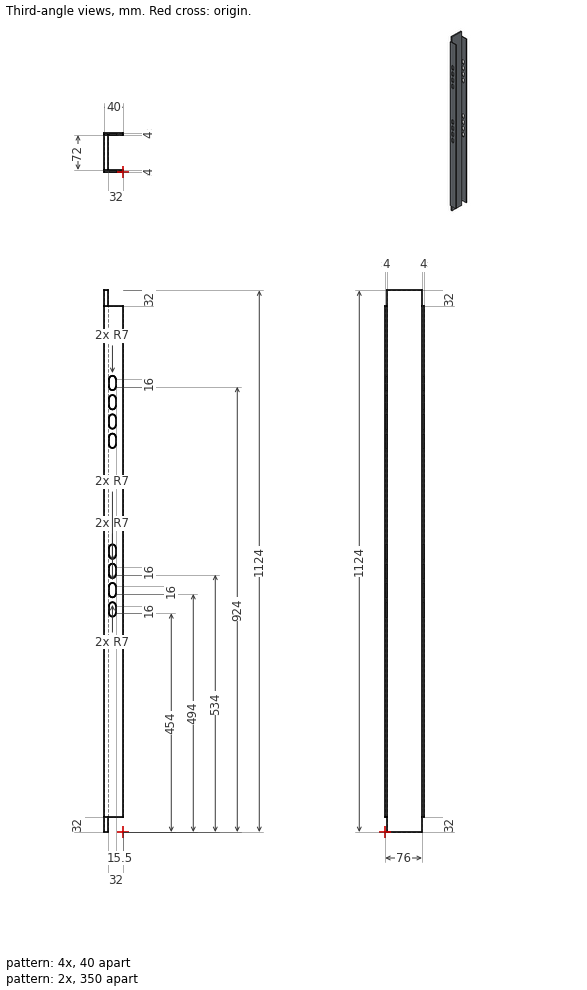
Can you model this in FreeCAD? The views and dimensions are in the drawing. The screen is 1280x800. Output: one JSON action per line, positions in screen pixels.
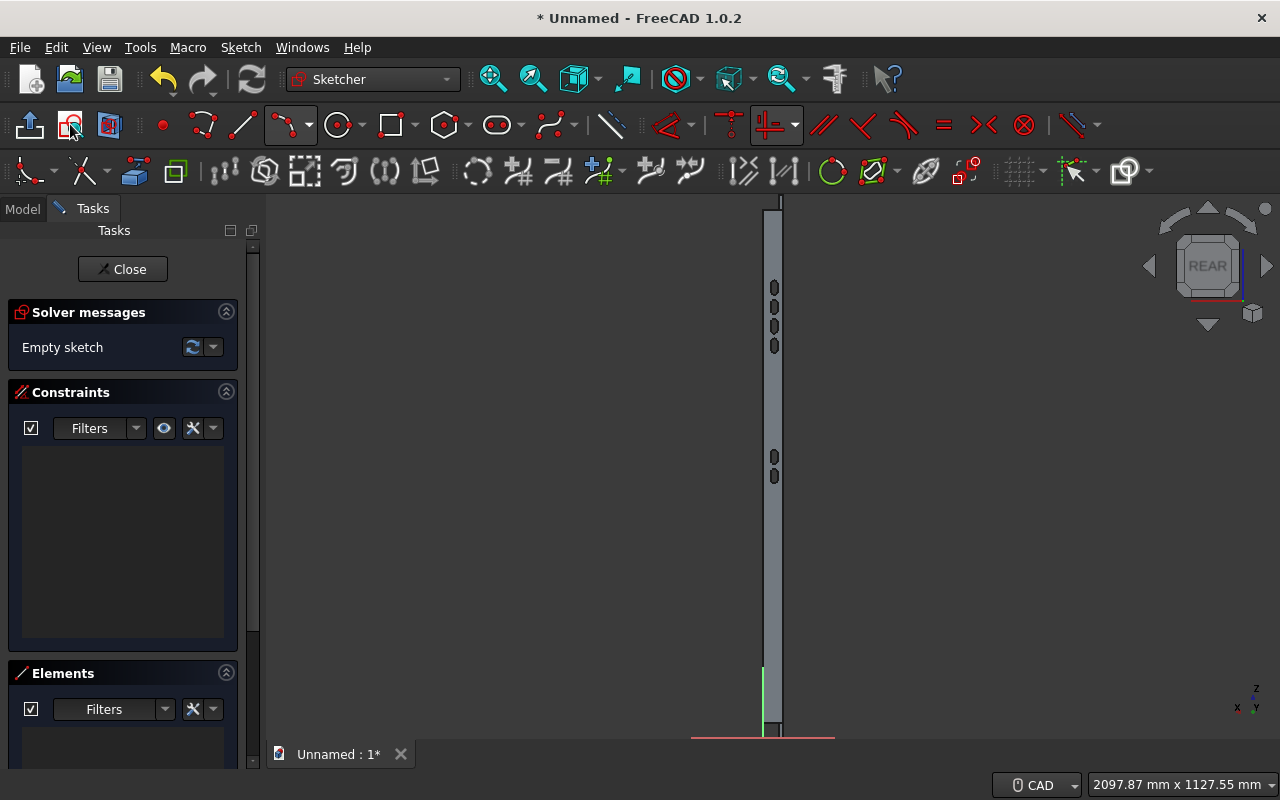
{"action": "scroll", "coordinate": [778, 497], "scroll_direction": "up", "scroll_amount": 15}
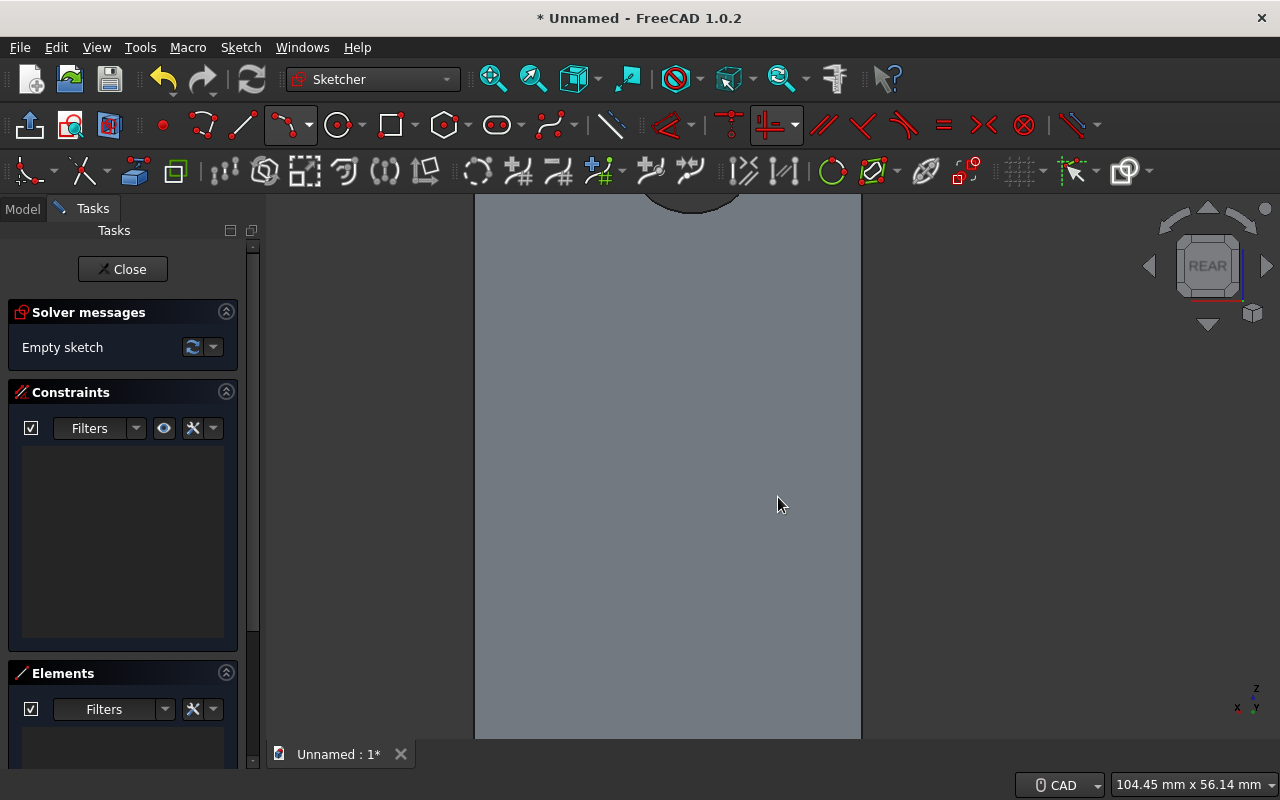
{"action": "left_click", "coordinate": [498, 126]}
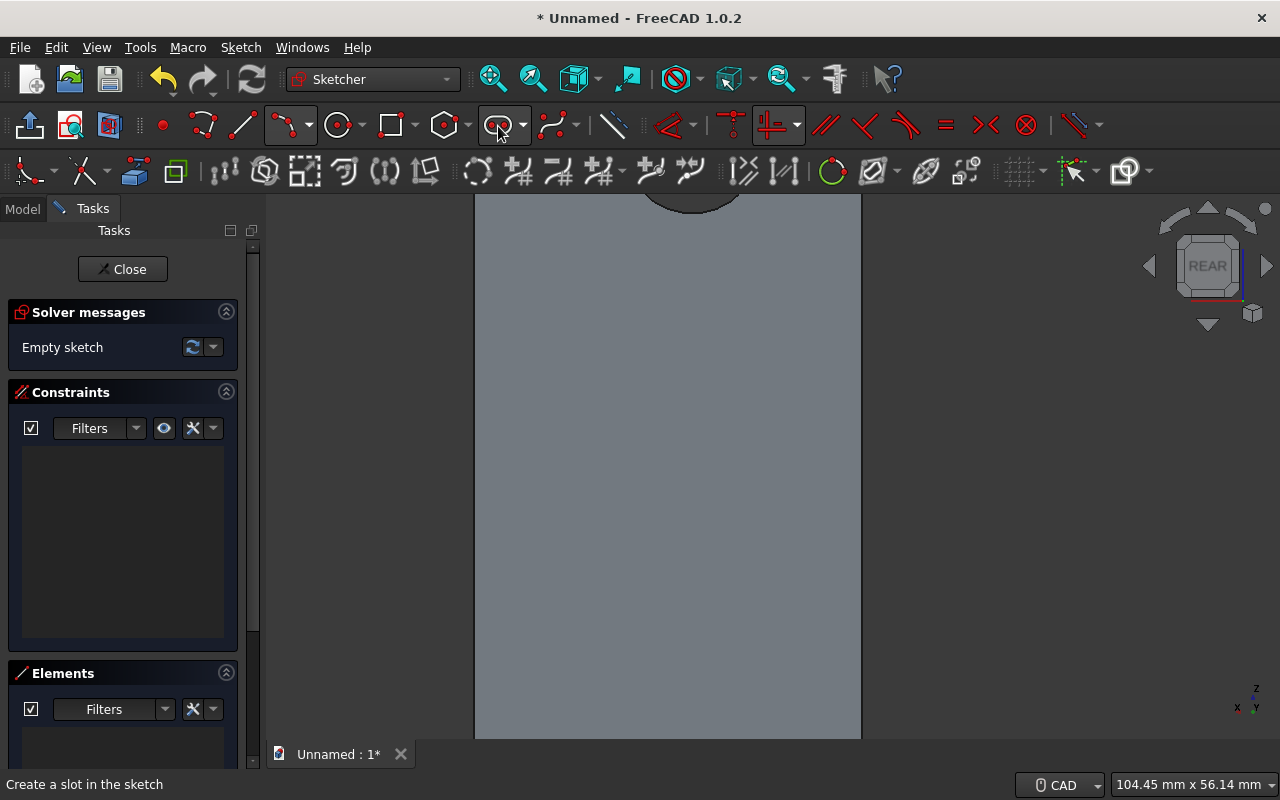
{"action": "left_click", "coordinate": [692, 534]}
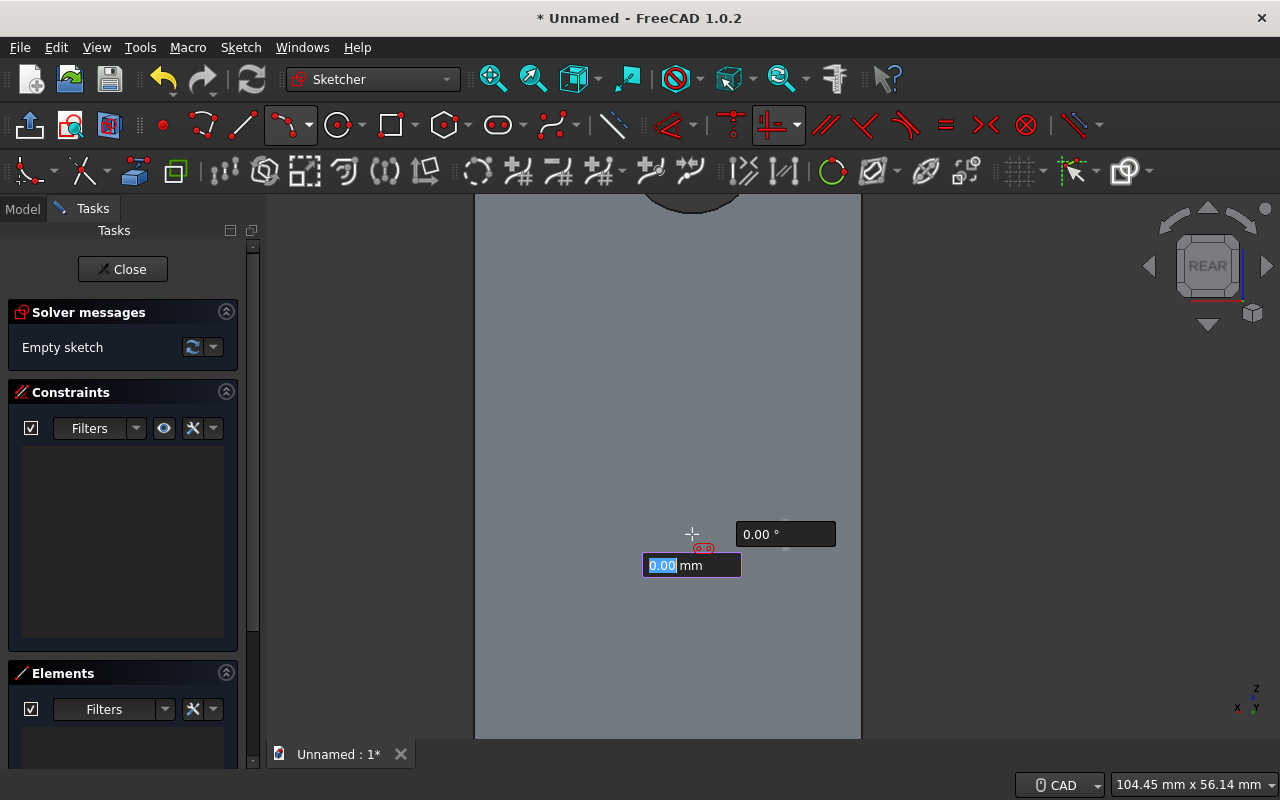
{"action": "left_click", "coordinate": [692, 379]}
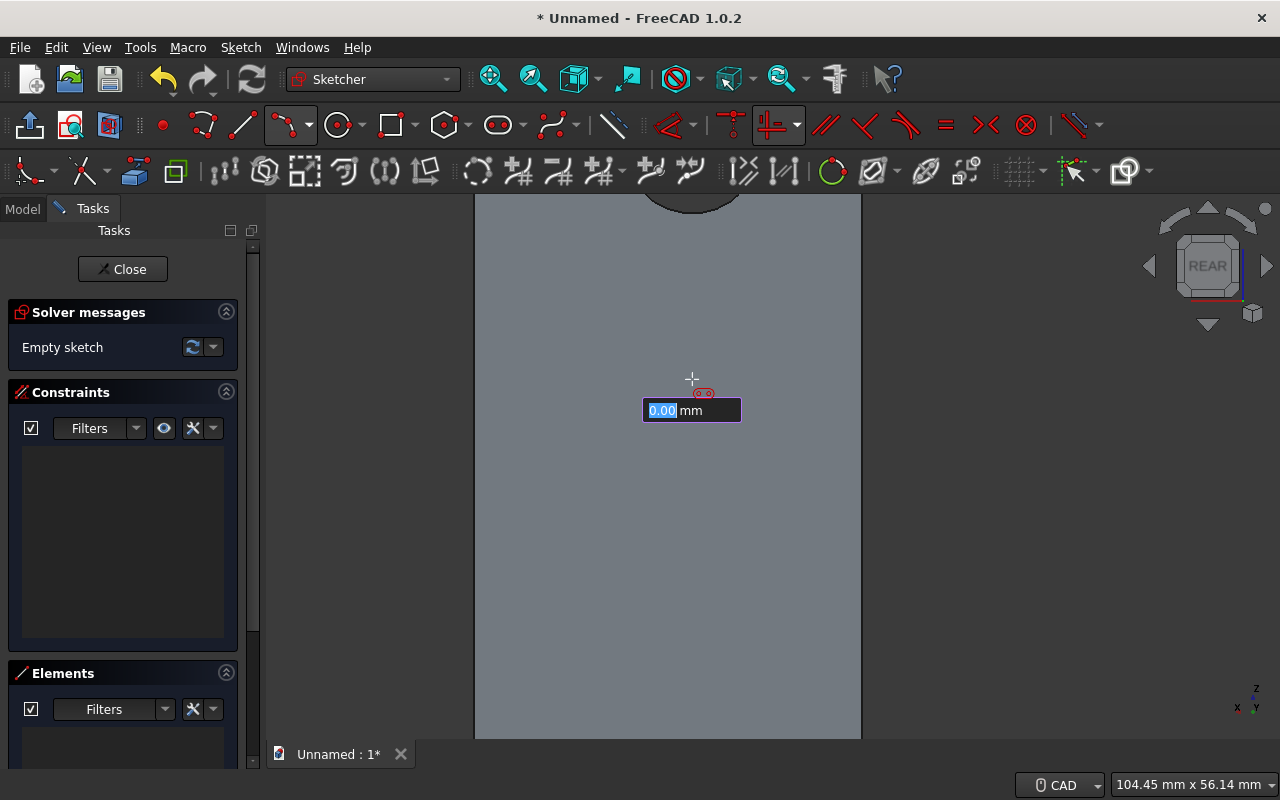
{"action": "left_click", "coordinate": [760, 456]}
{"action": "key", "text": "Escape"}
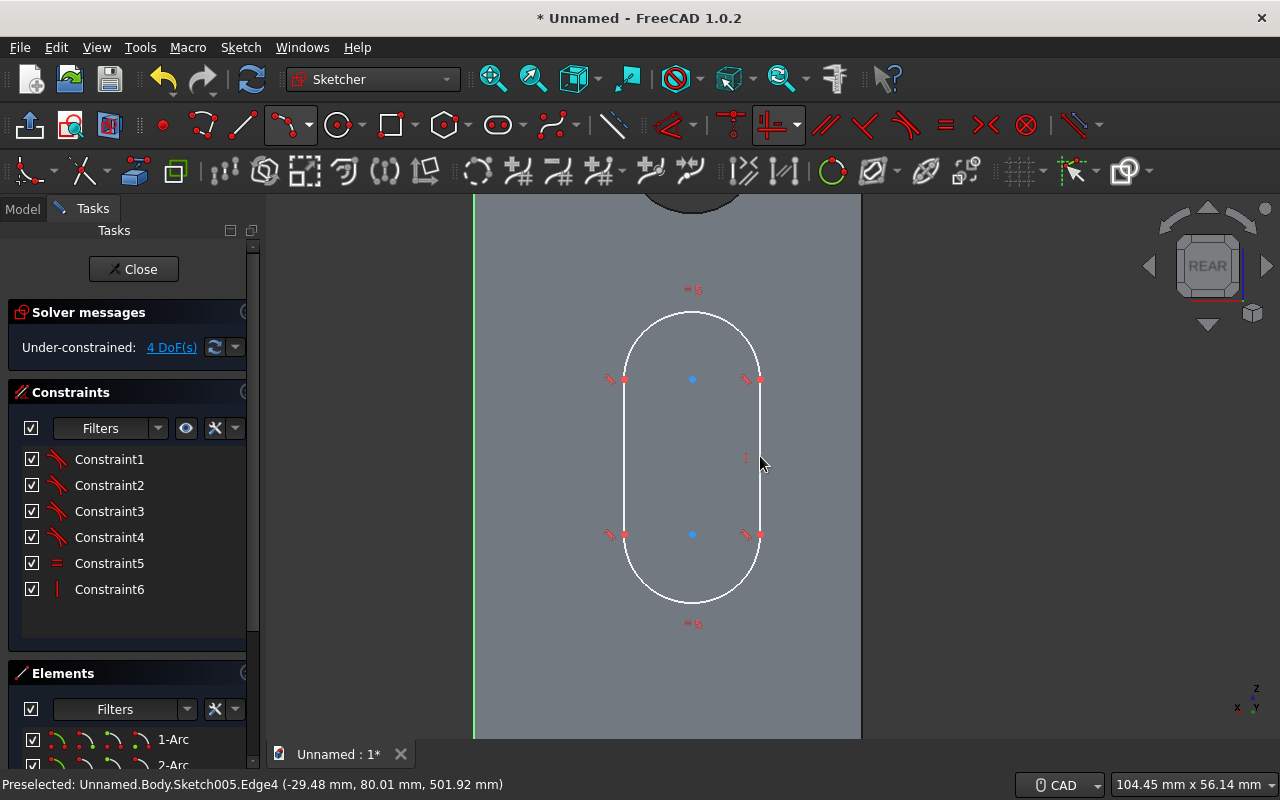
{"action": "left_click", "coordinate": [668, 126]}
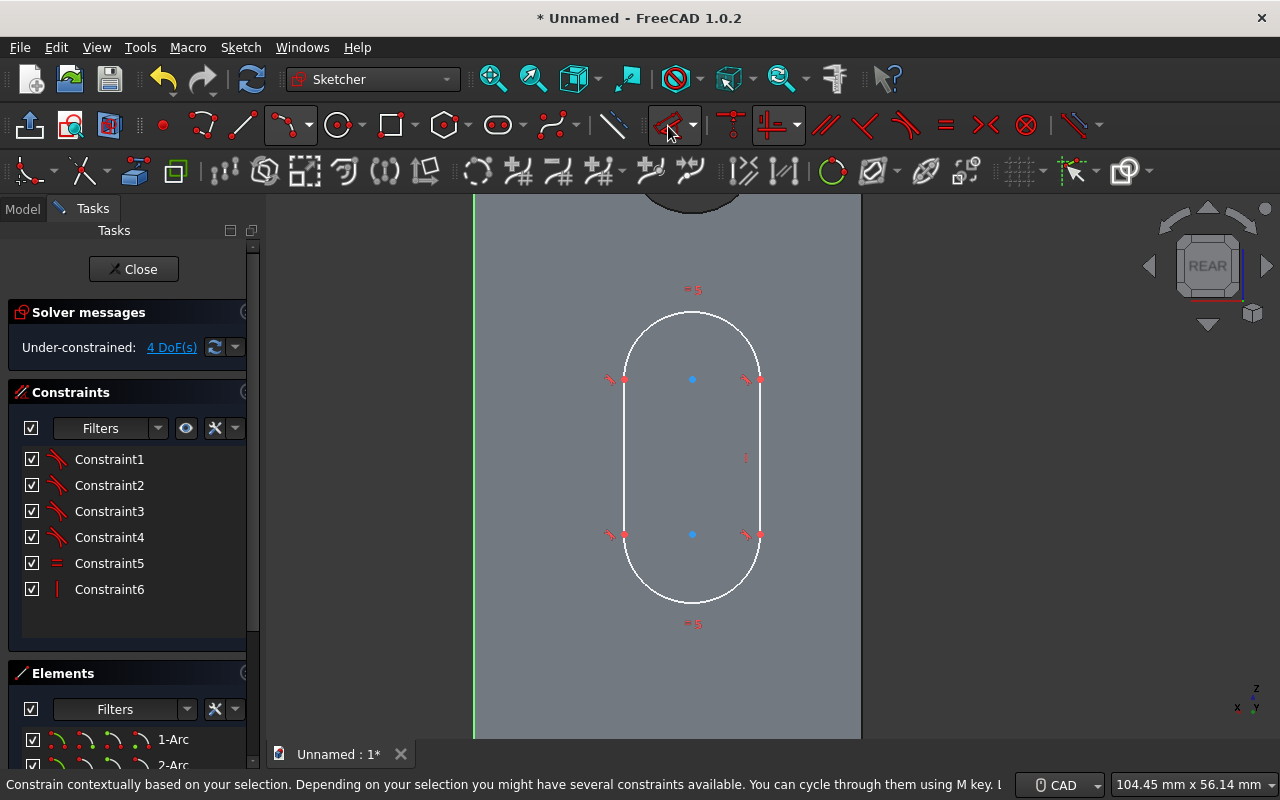
{"action": "left_click", "coordinate": [652, 590]}
{"action": "left_click", "coordinate": [633, 616]}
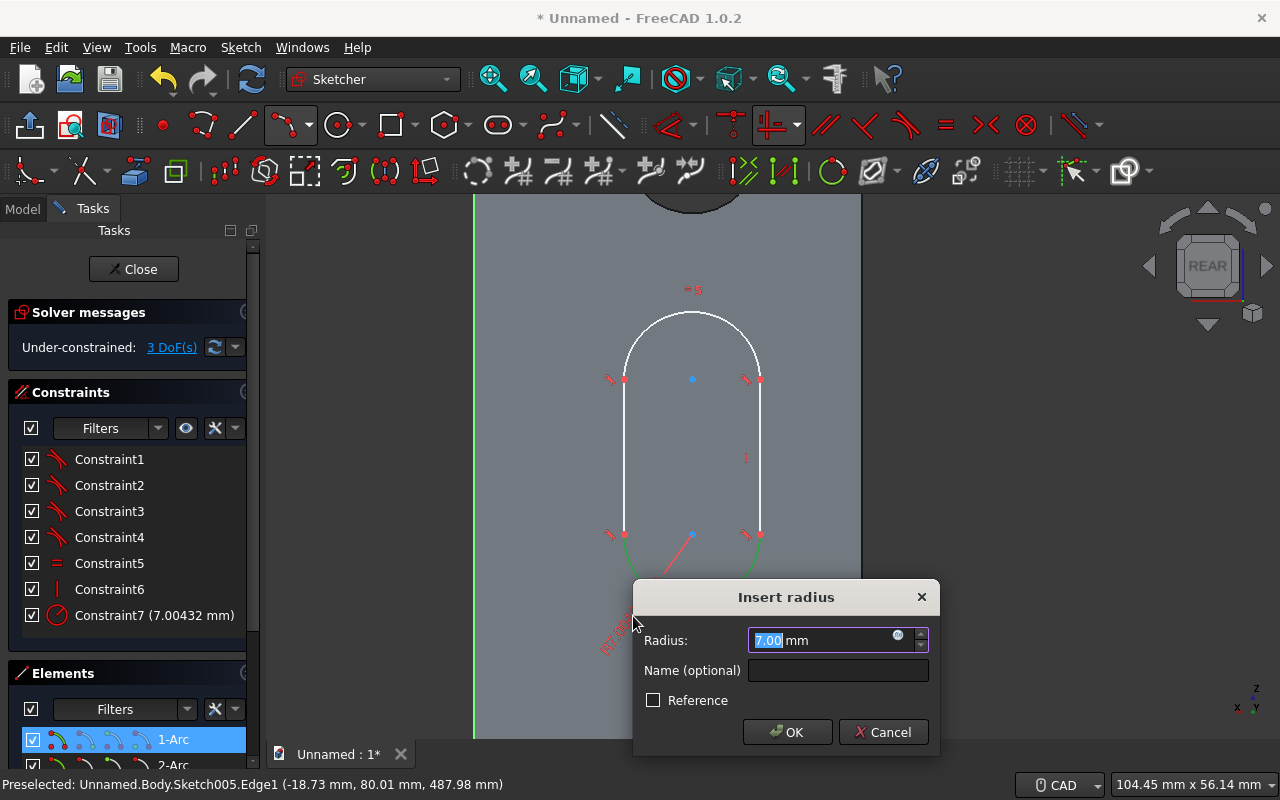
{"action": "type", "text": "7"}
{"action": "key", "text": "Return"}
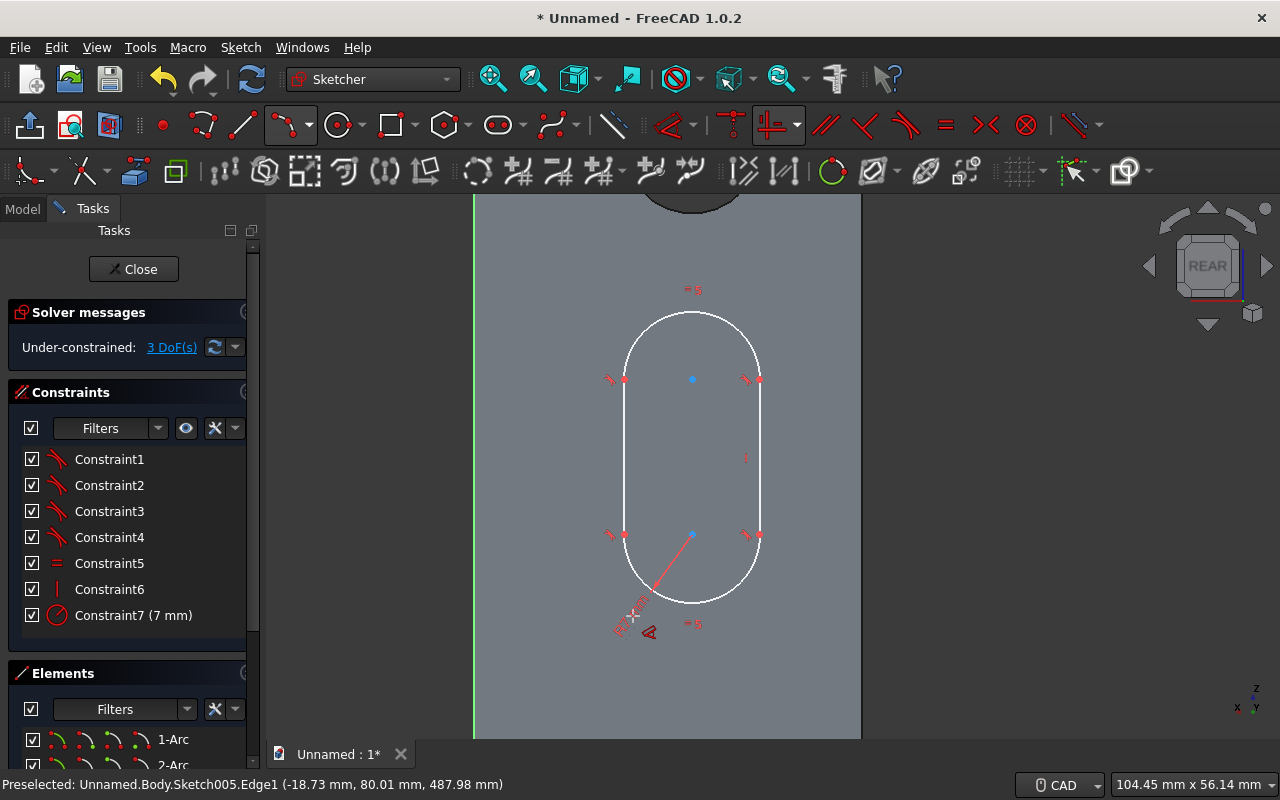
{"action": "left_click", "coordinate": [624, 488]}
{"action": "left_click", "coordinate": [590, 457]}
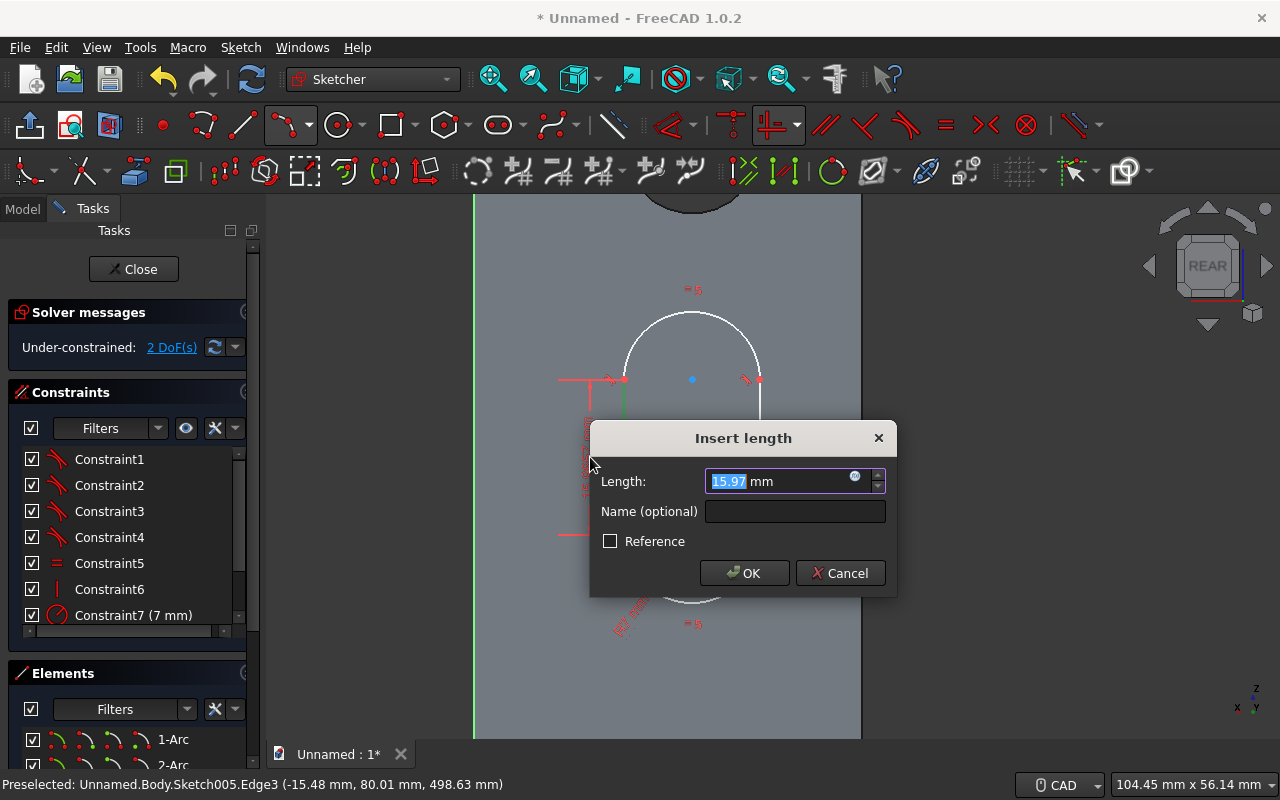
{"action": "type", "text": "16"}
{"action": "key", "text": "Return"}